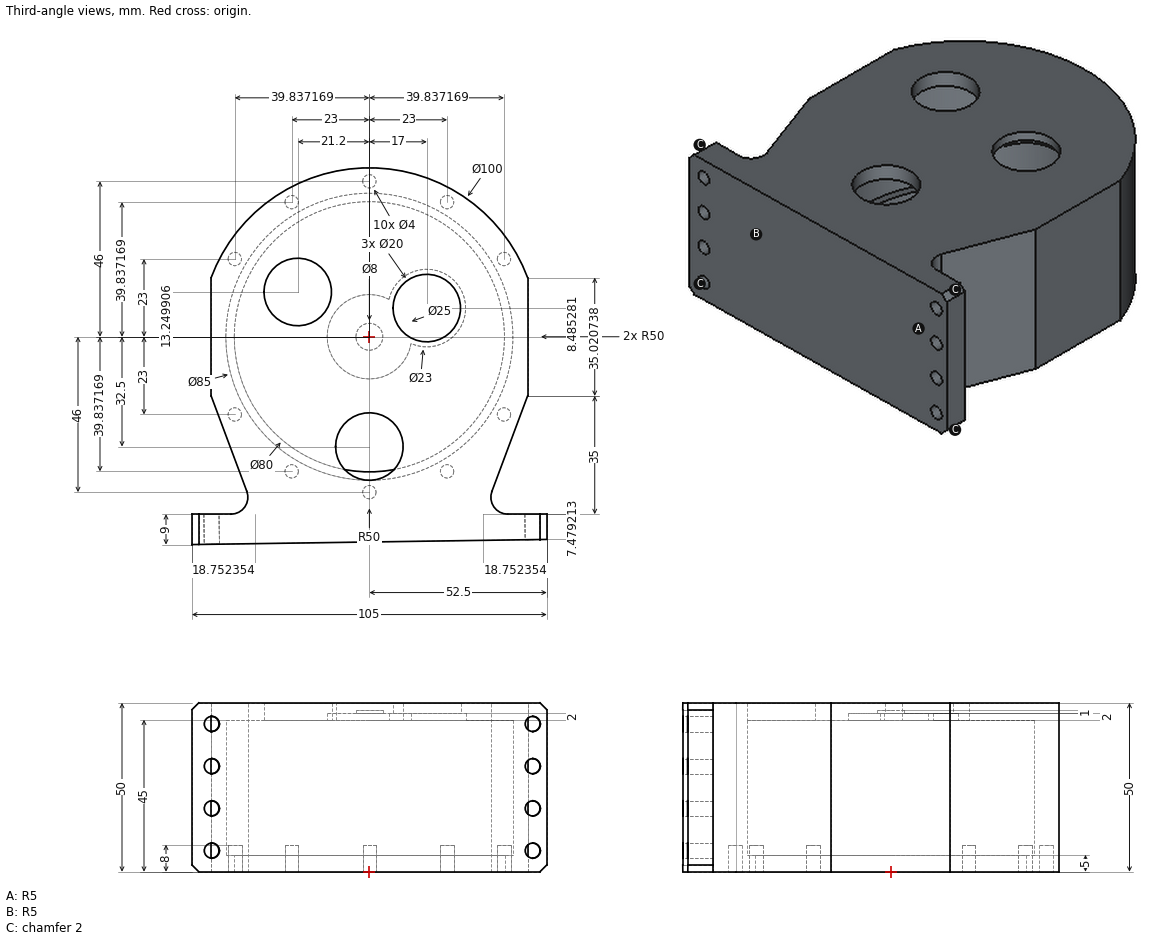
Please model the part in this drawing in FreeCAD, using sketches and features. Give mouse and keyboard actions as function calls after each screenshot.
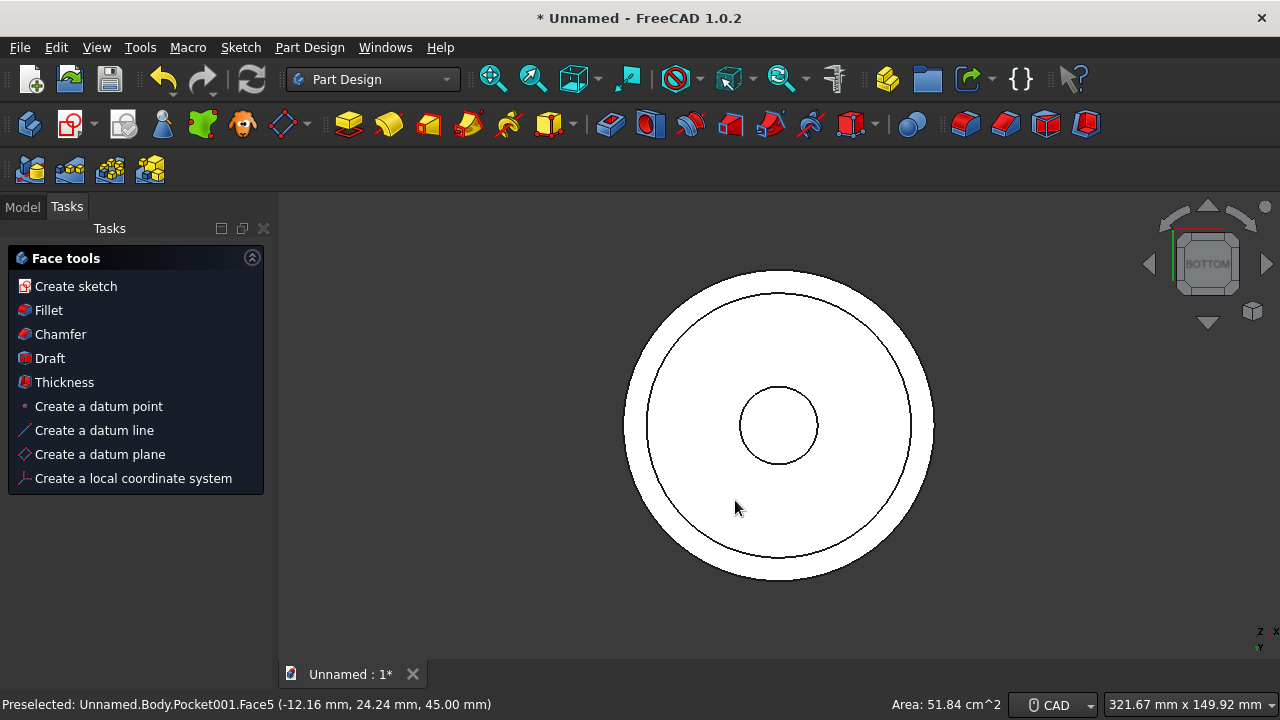
click(70, 124)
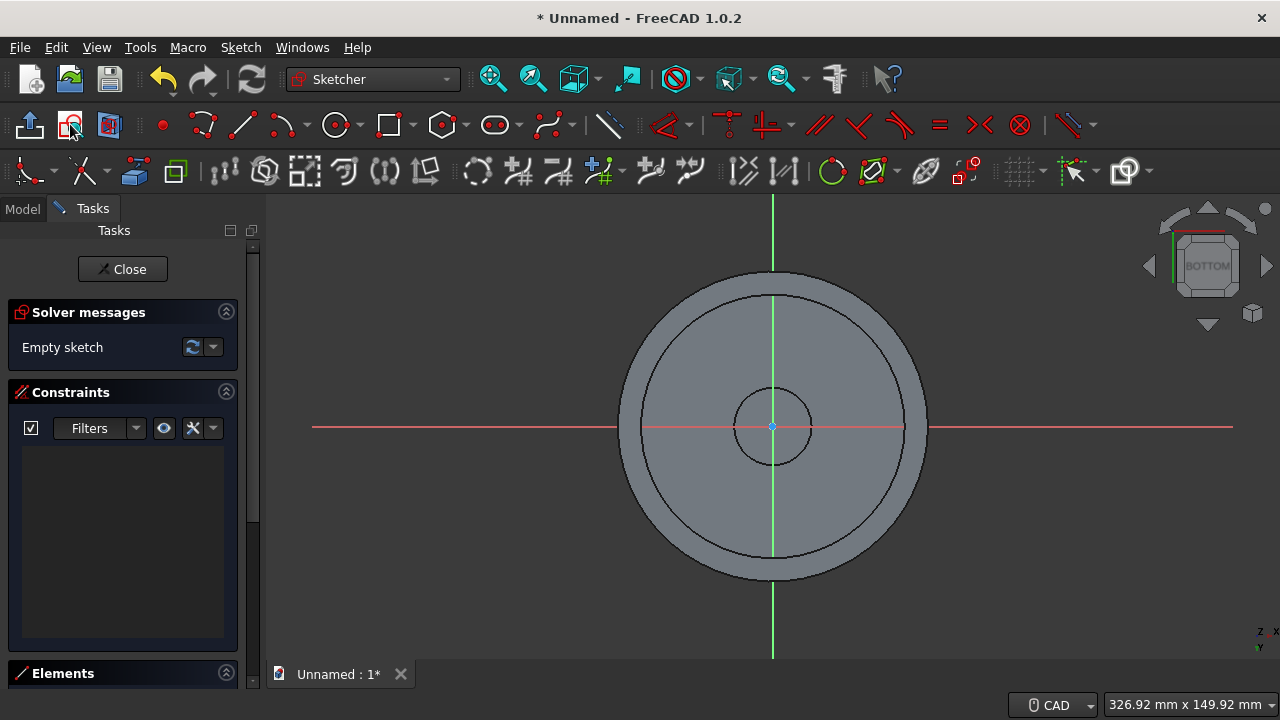
key(q)
key(s)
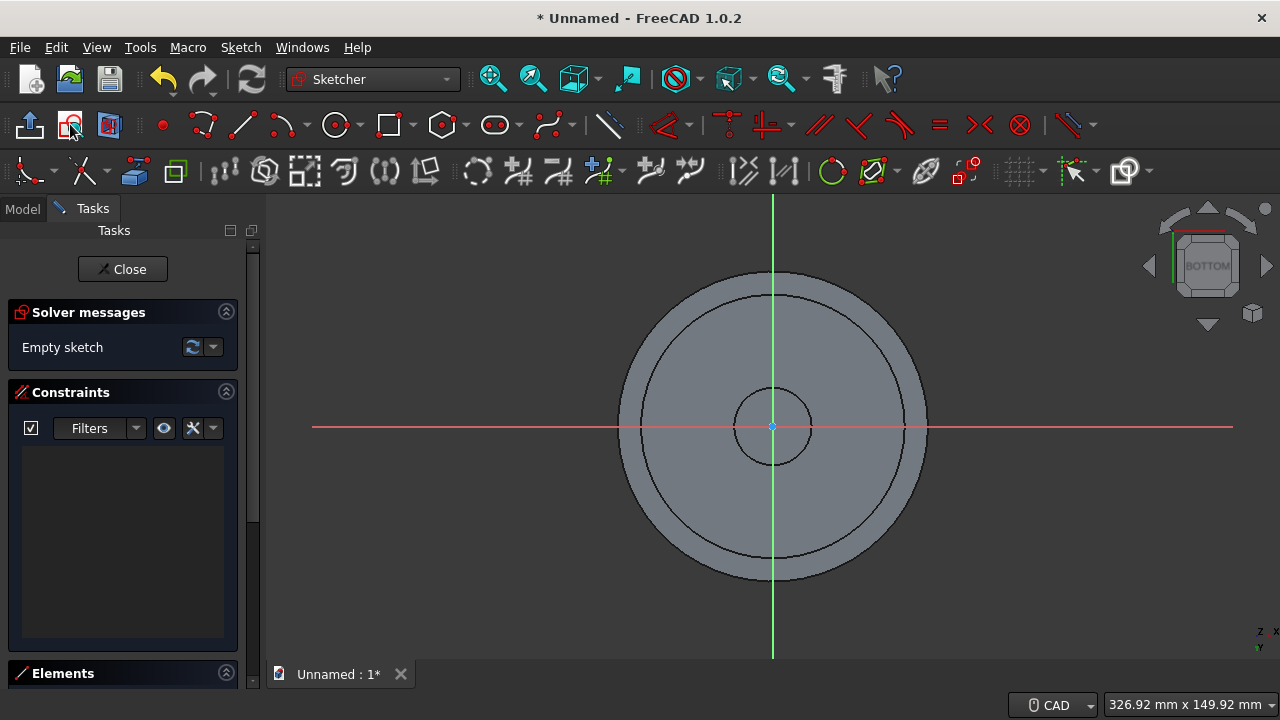
scroll(892, 336, up, 2)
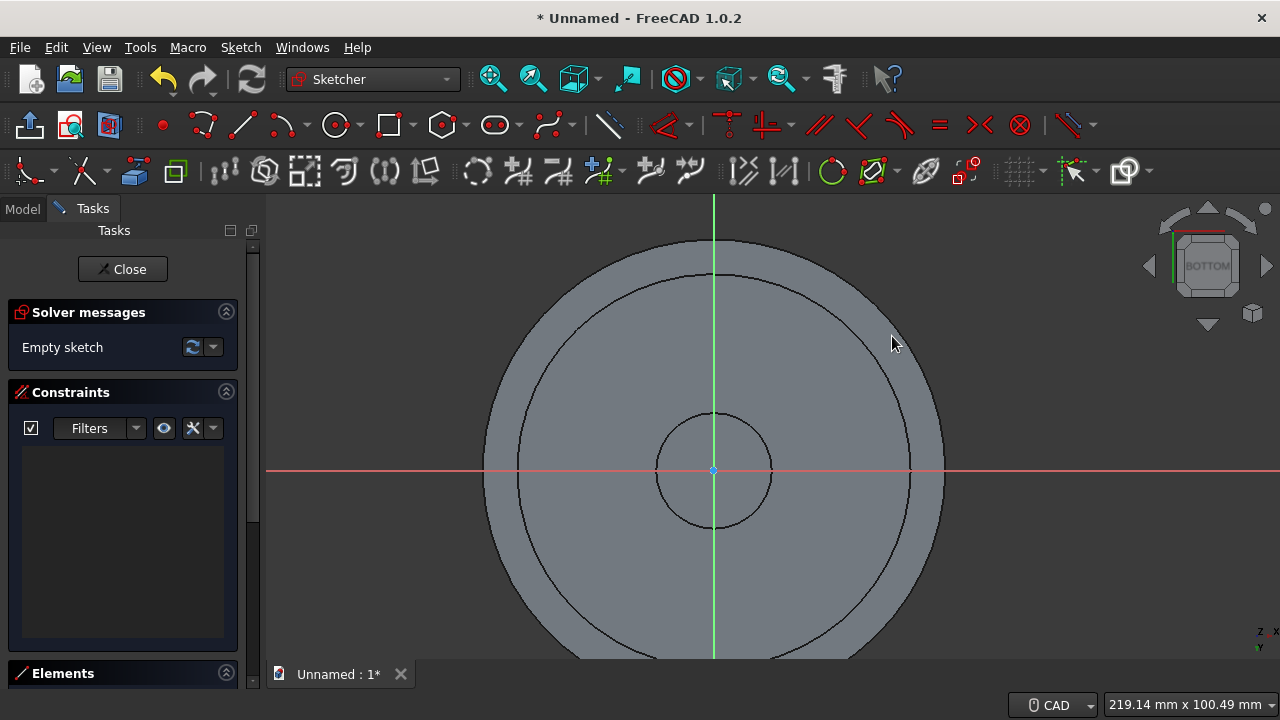
click(336, 126)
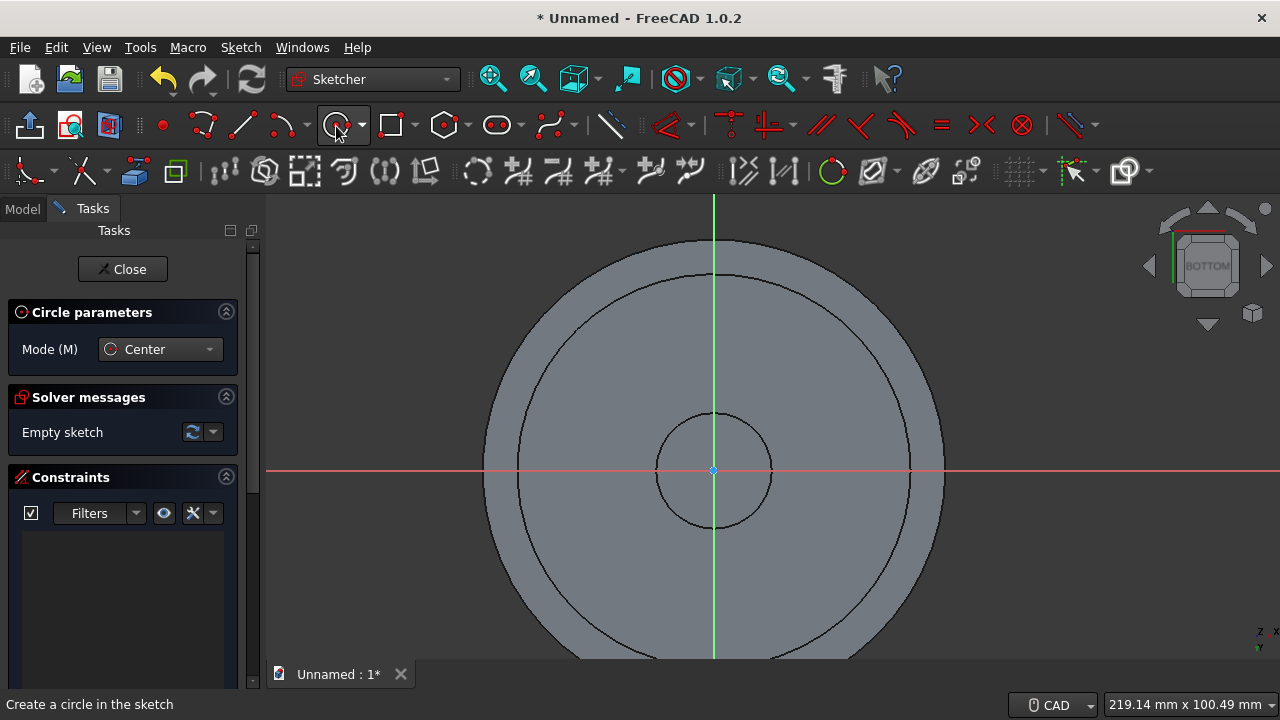
click(793, 510)
click(825, 543)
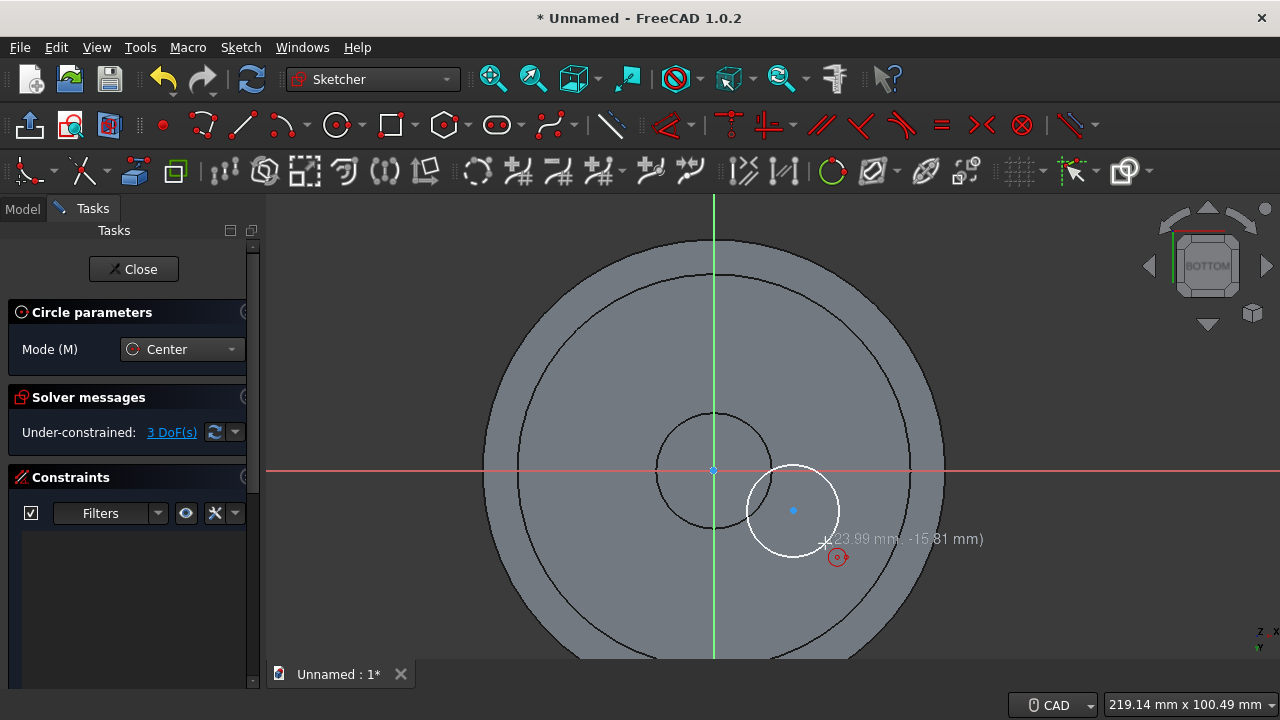
click(616, 532)
click(649, 499)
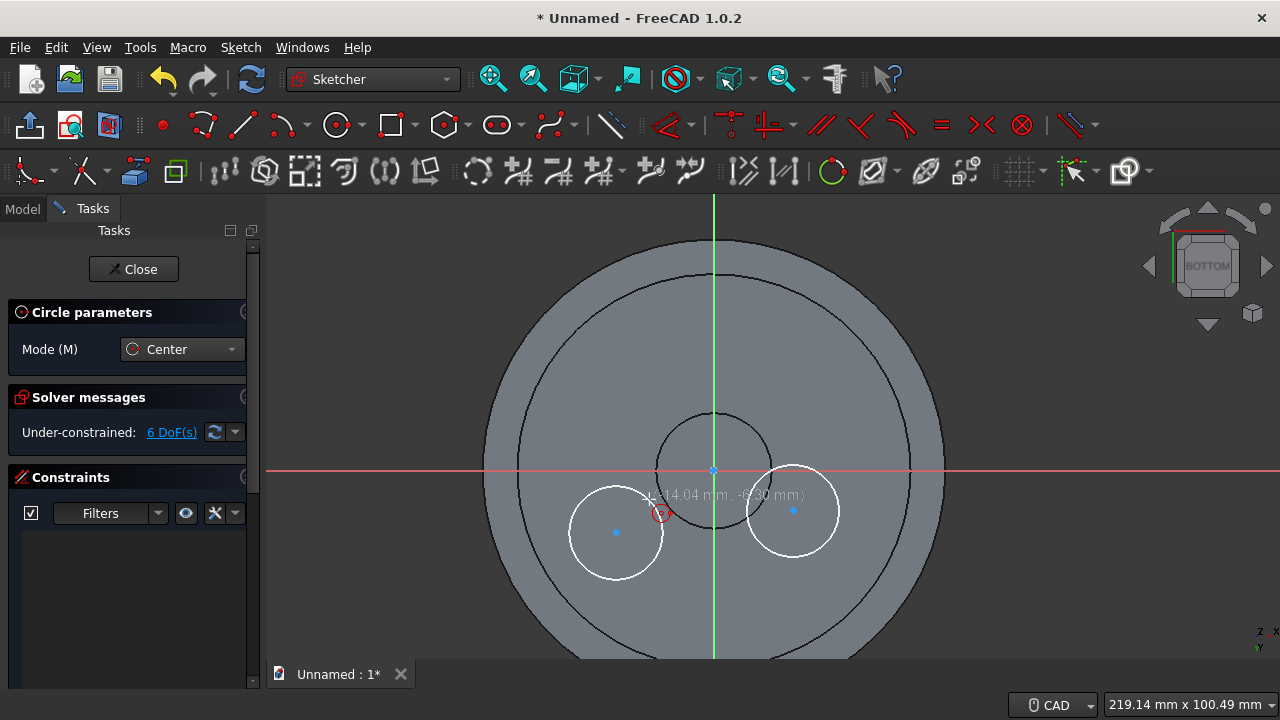
click(714, 320)
click(747, 288)
key(Escape)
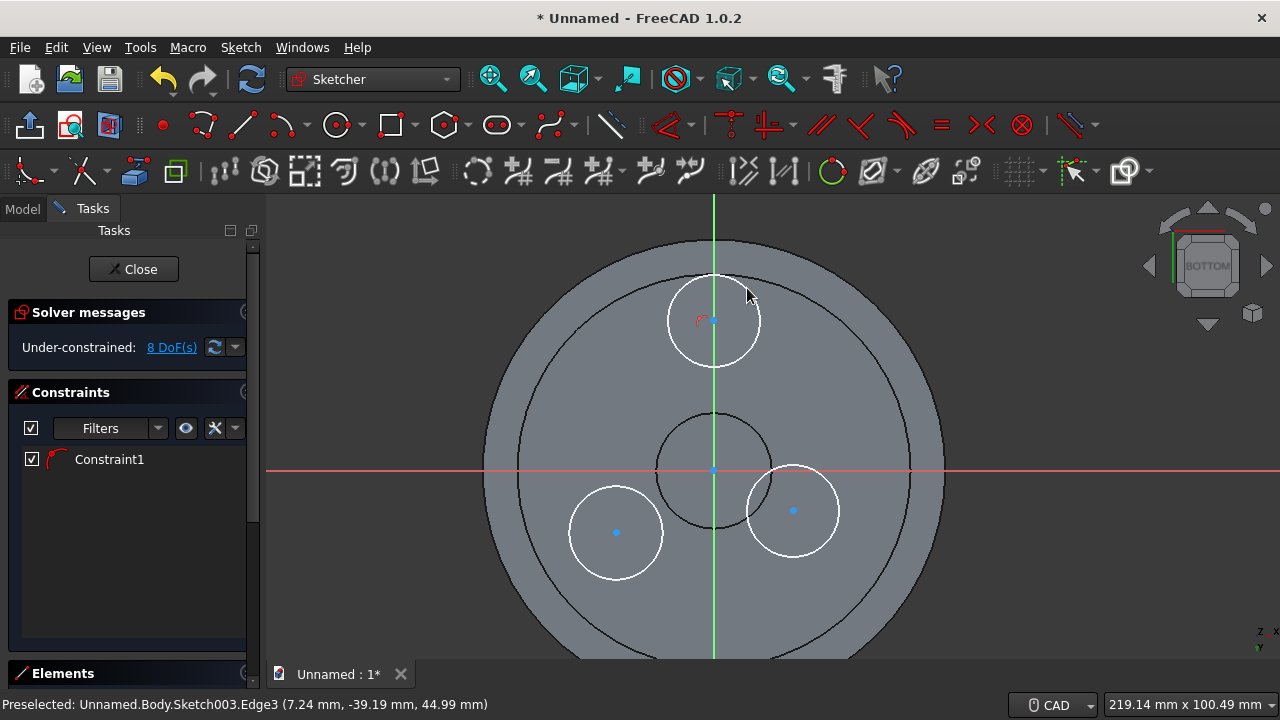
click(761, 544)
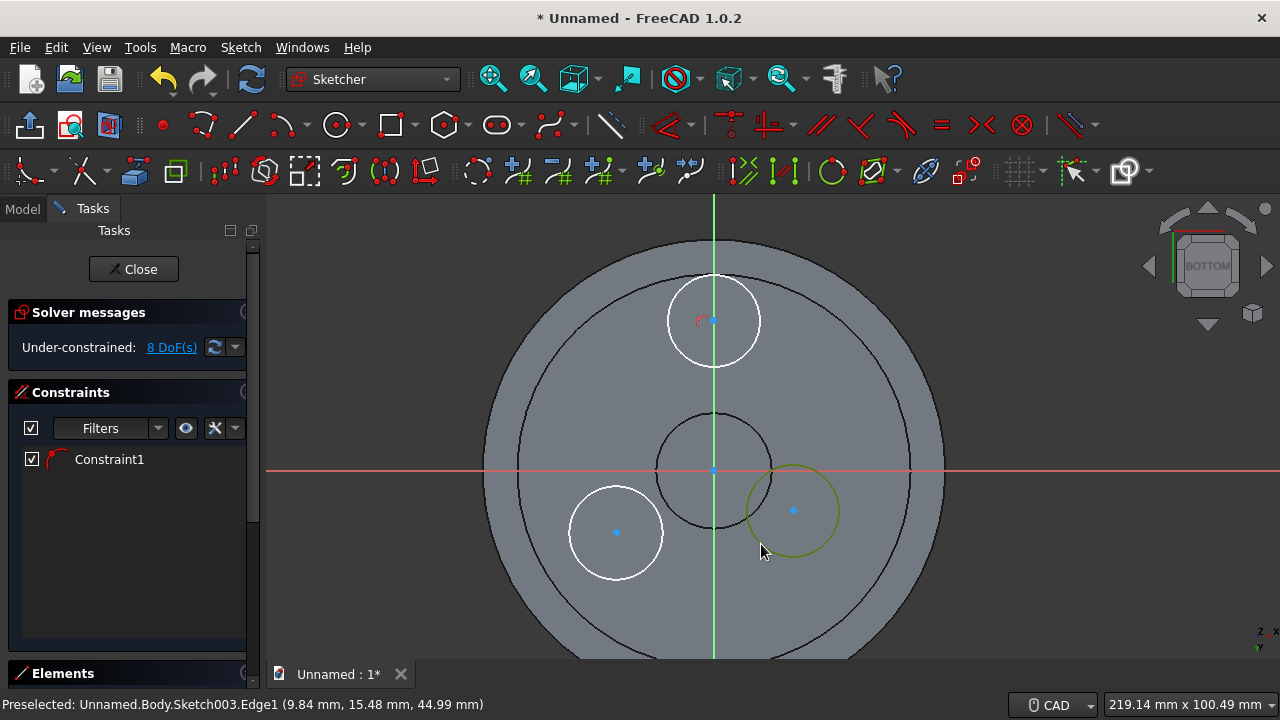
click(649, 500)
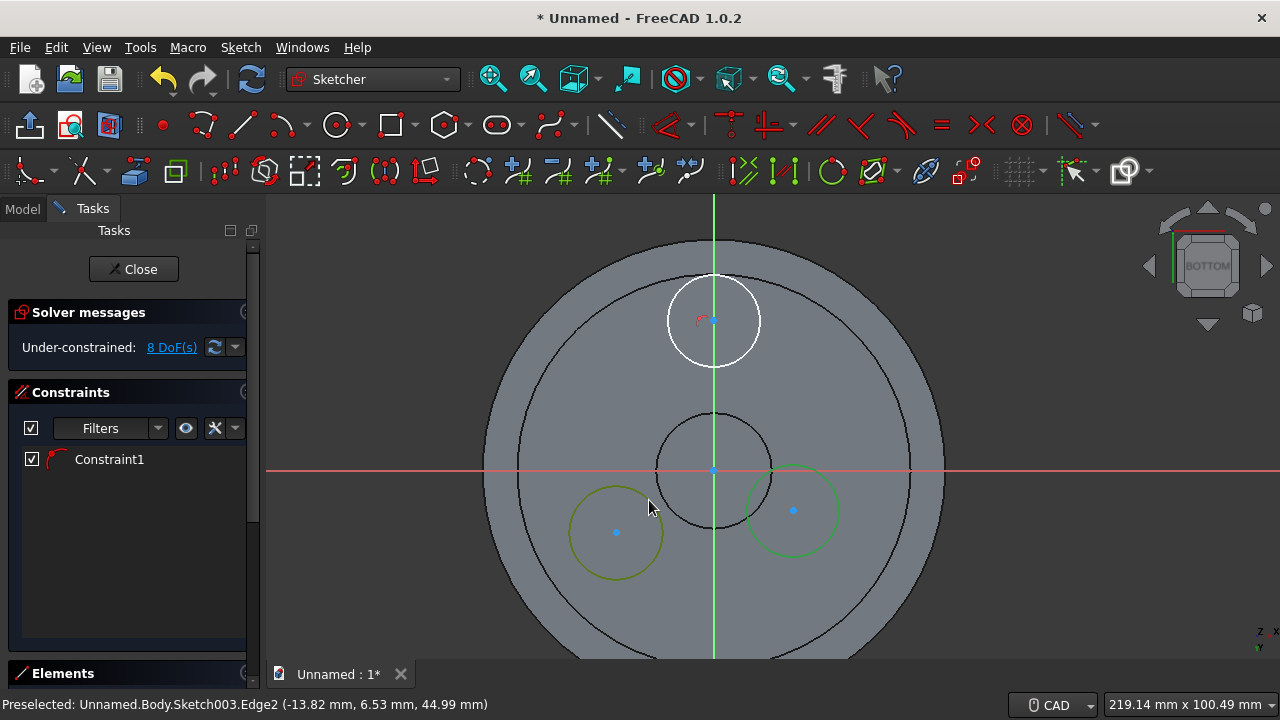
click(746, 288)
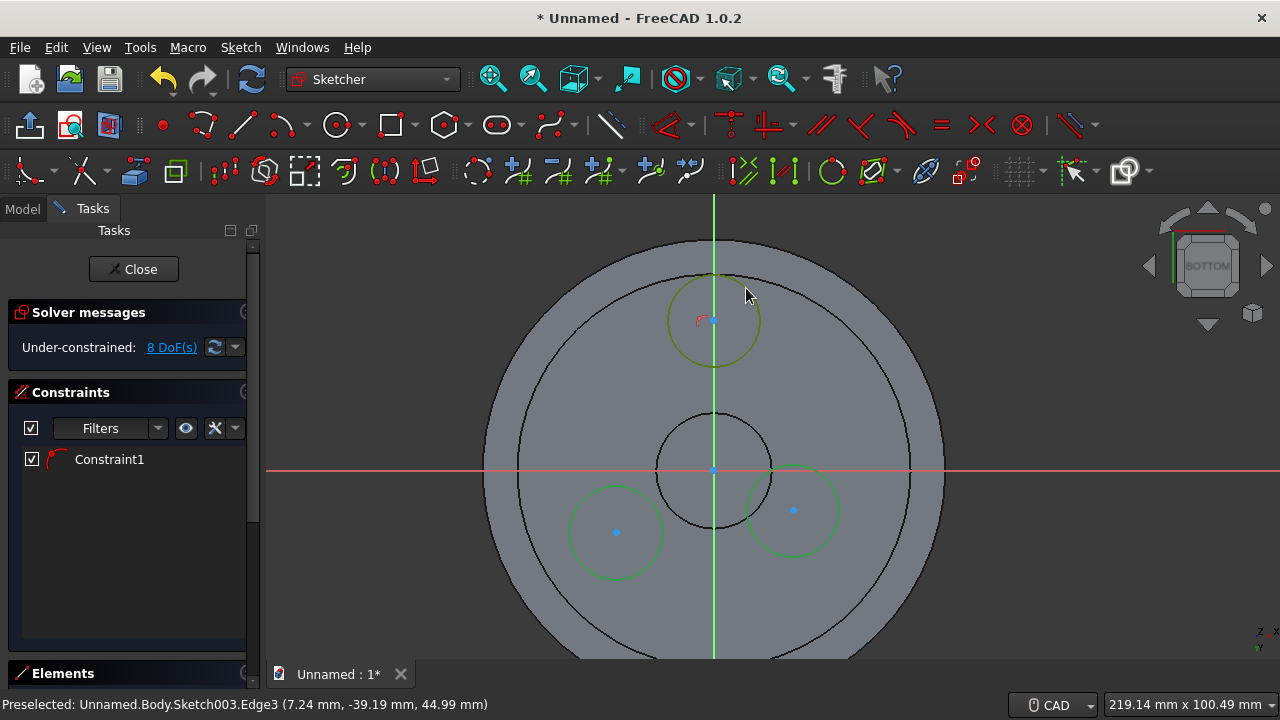
click(942, 126)